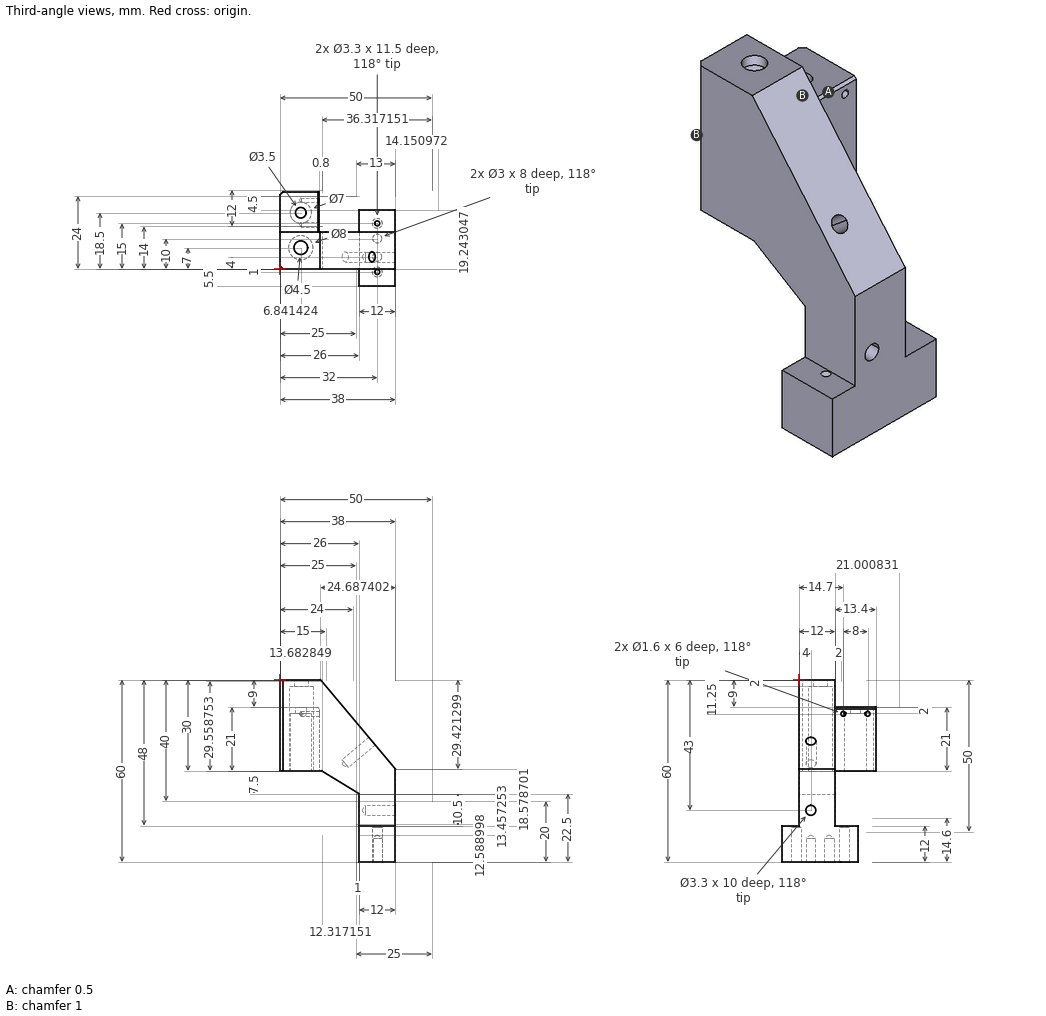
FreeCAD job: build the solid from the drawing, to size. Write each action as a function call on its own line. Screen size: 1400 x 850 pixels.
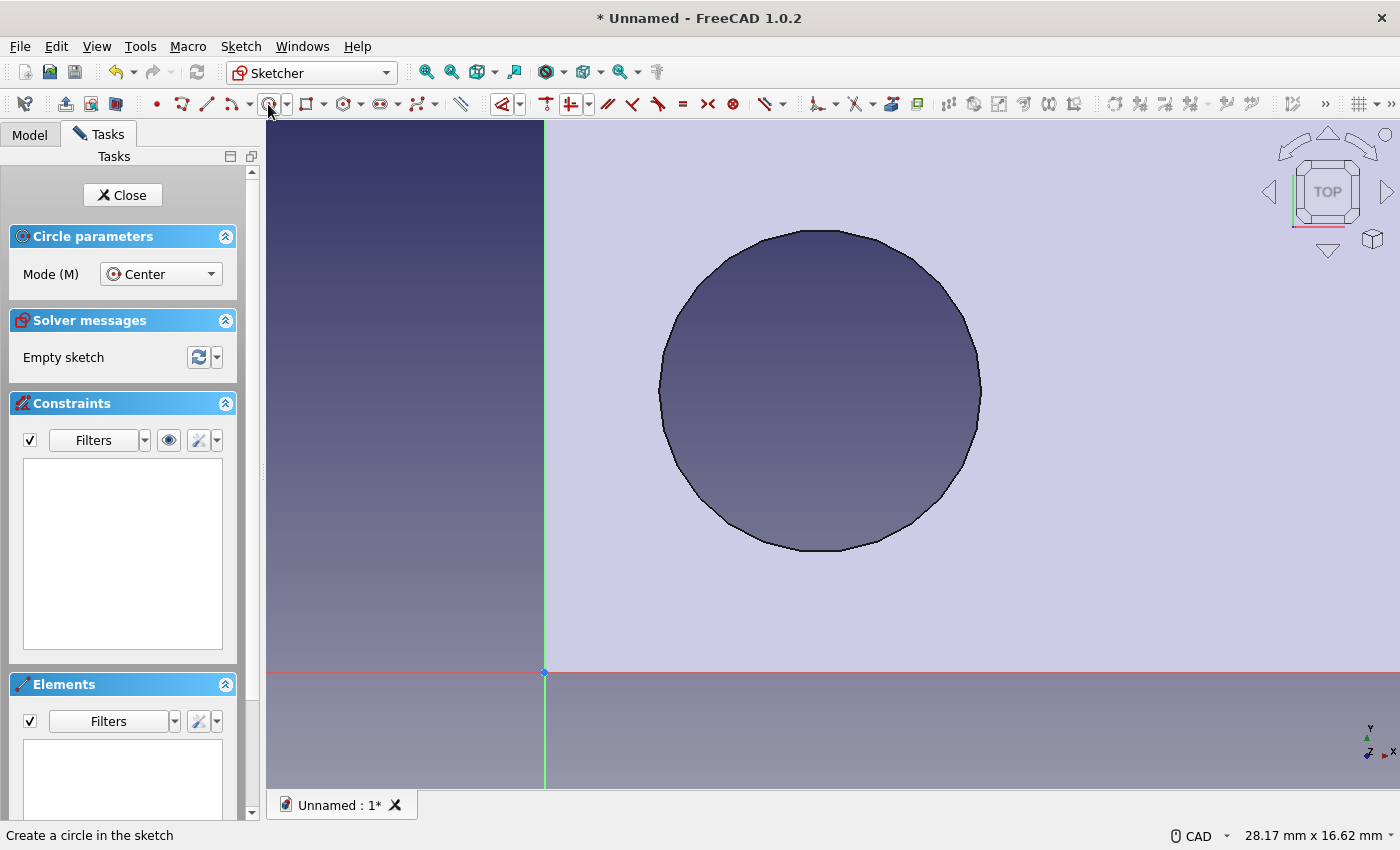
click(820, 391)
click(934, 277)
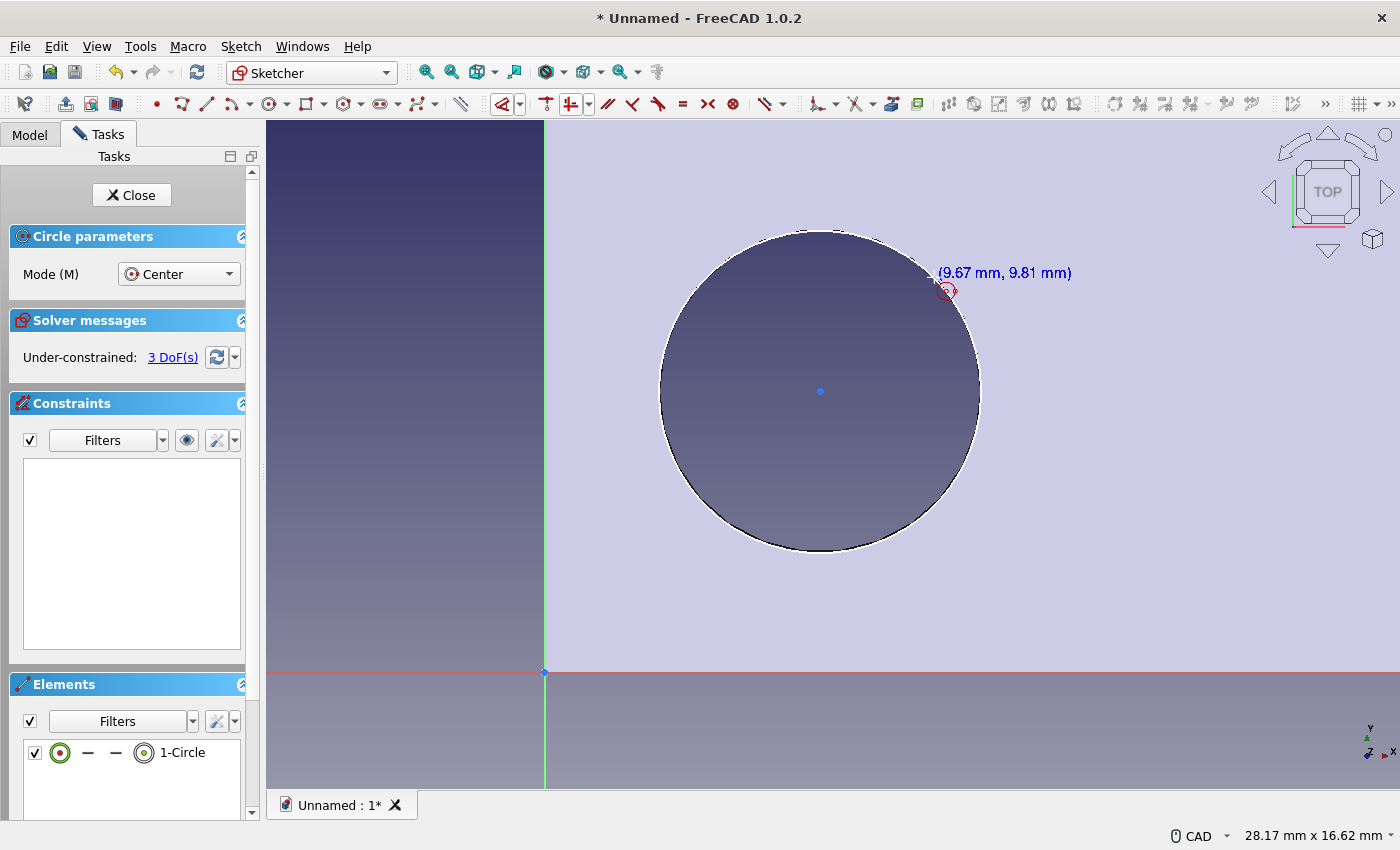
click(820, 392)
click(884, 327)
key(Escape)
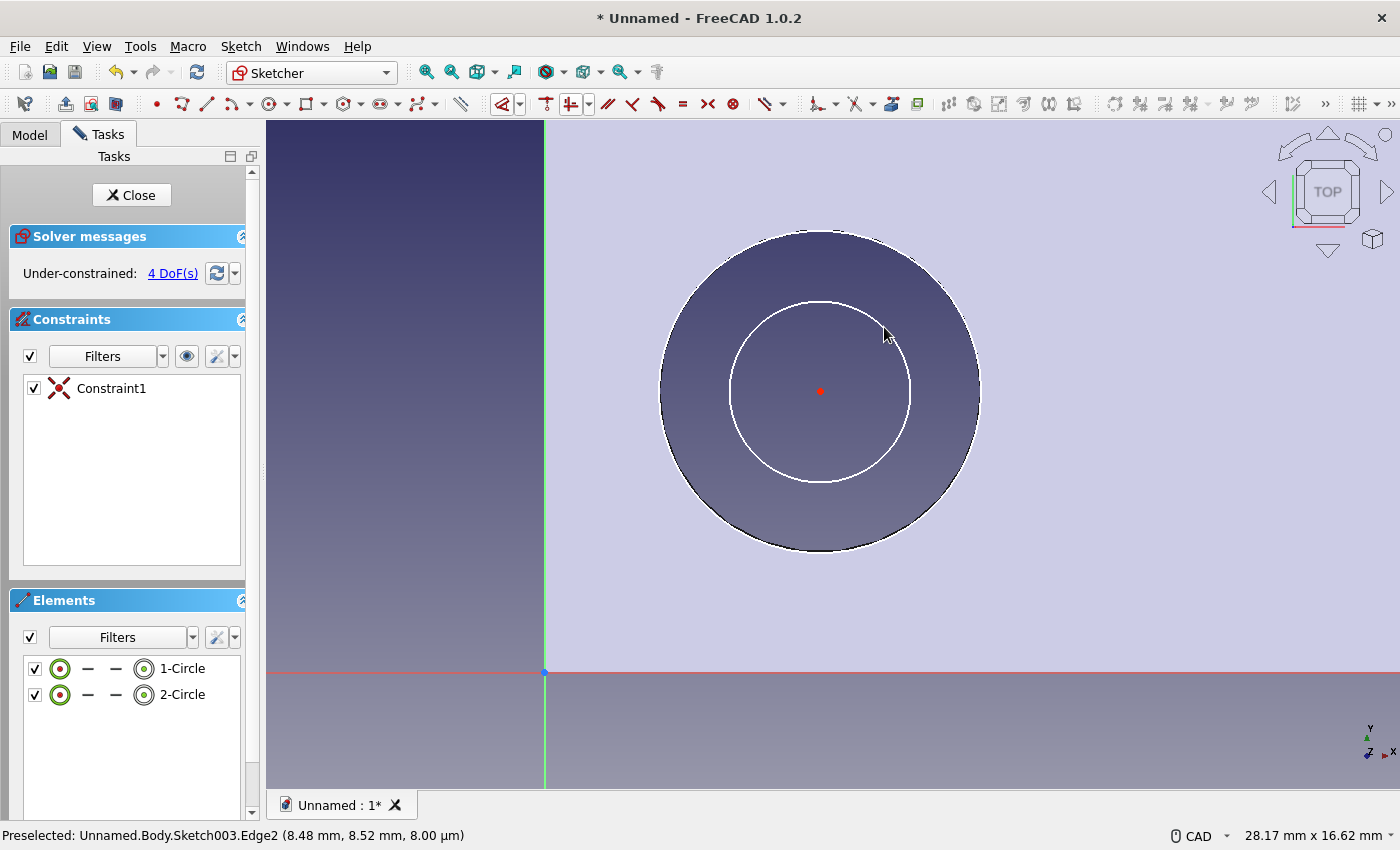
click(934, 278)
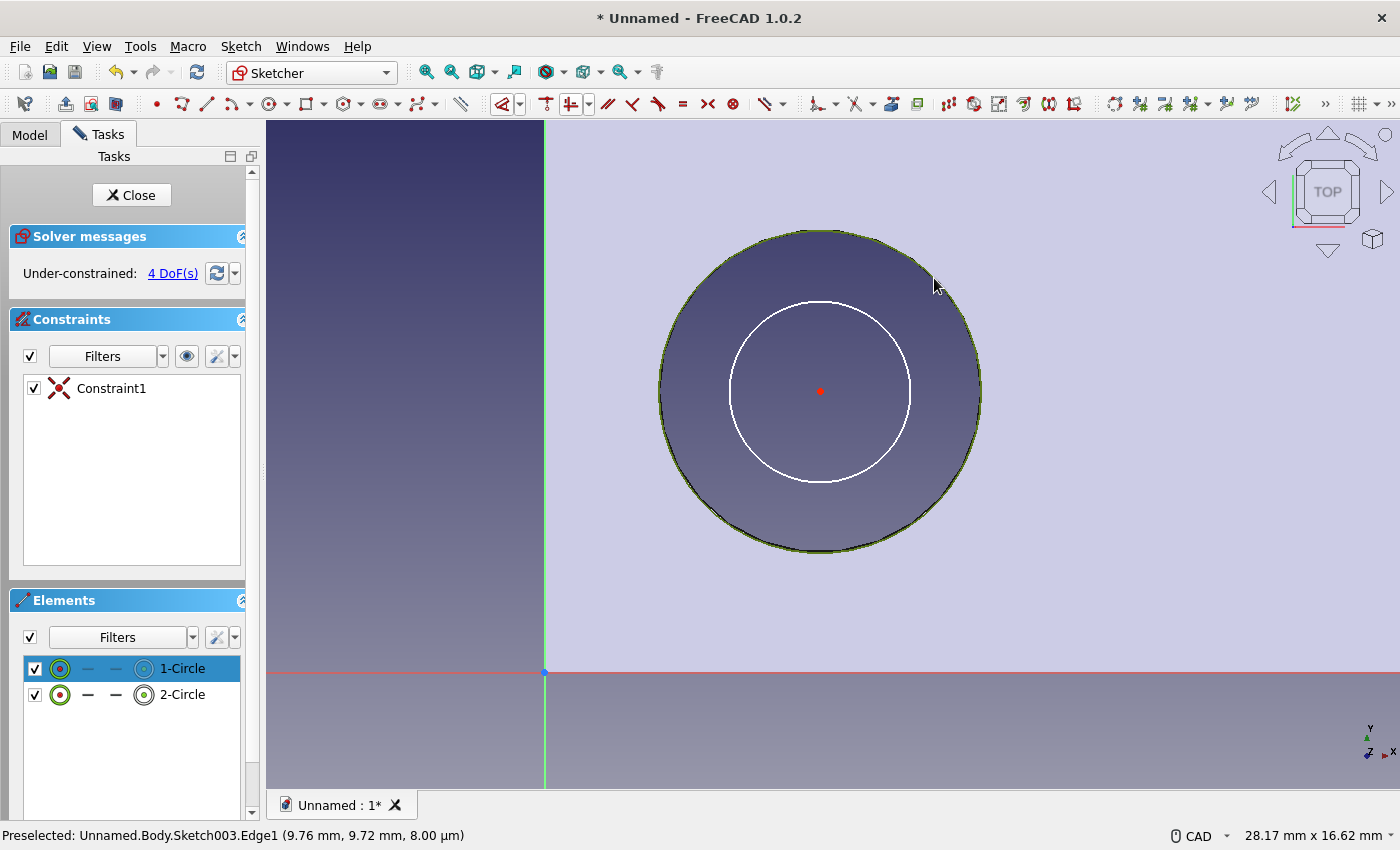
click(520, 104)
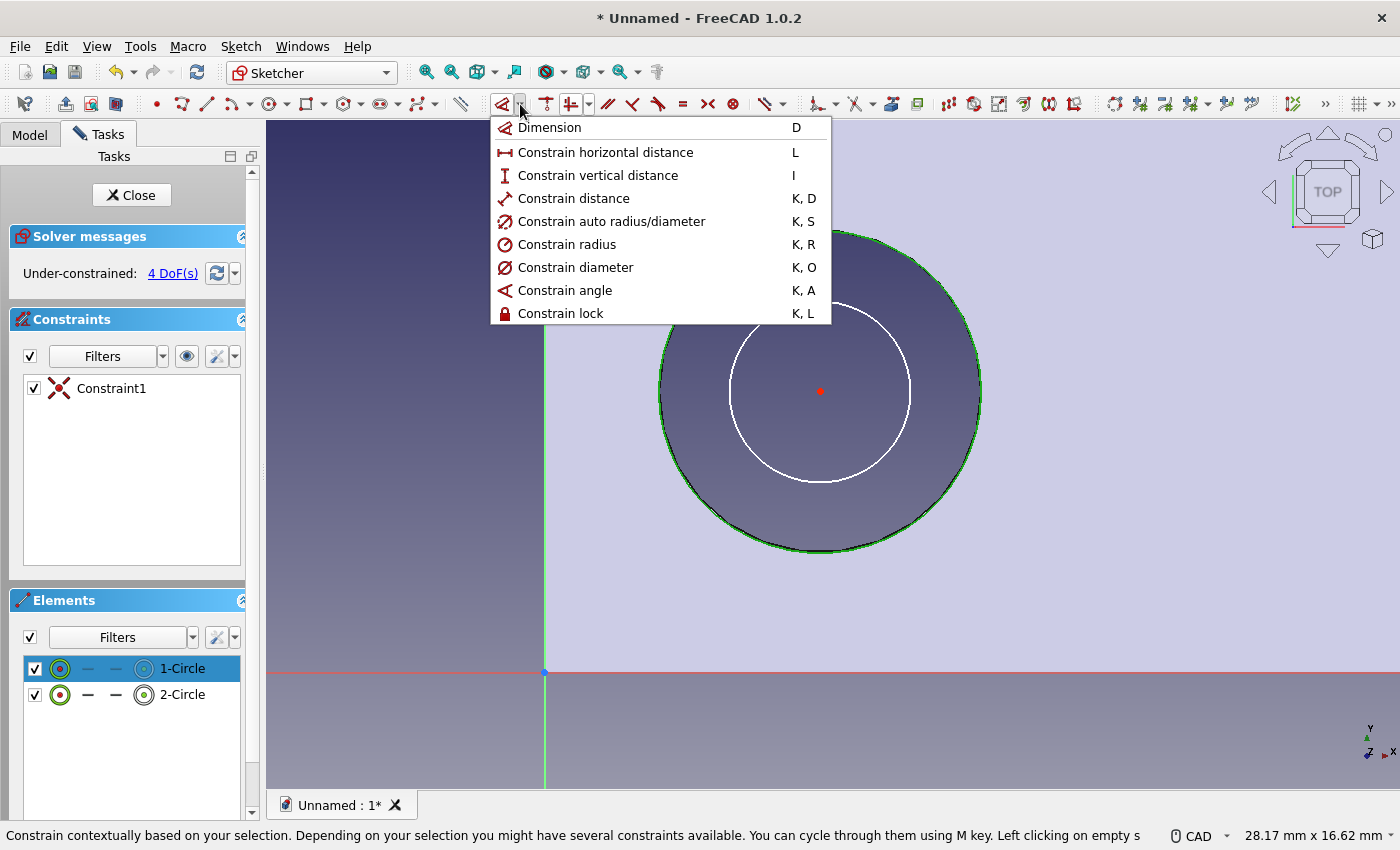
click(661, 268)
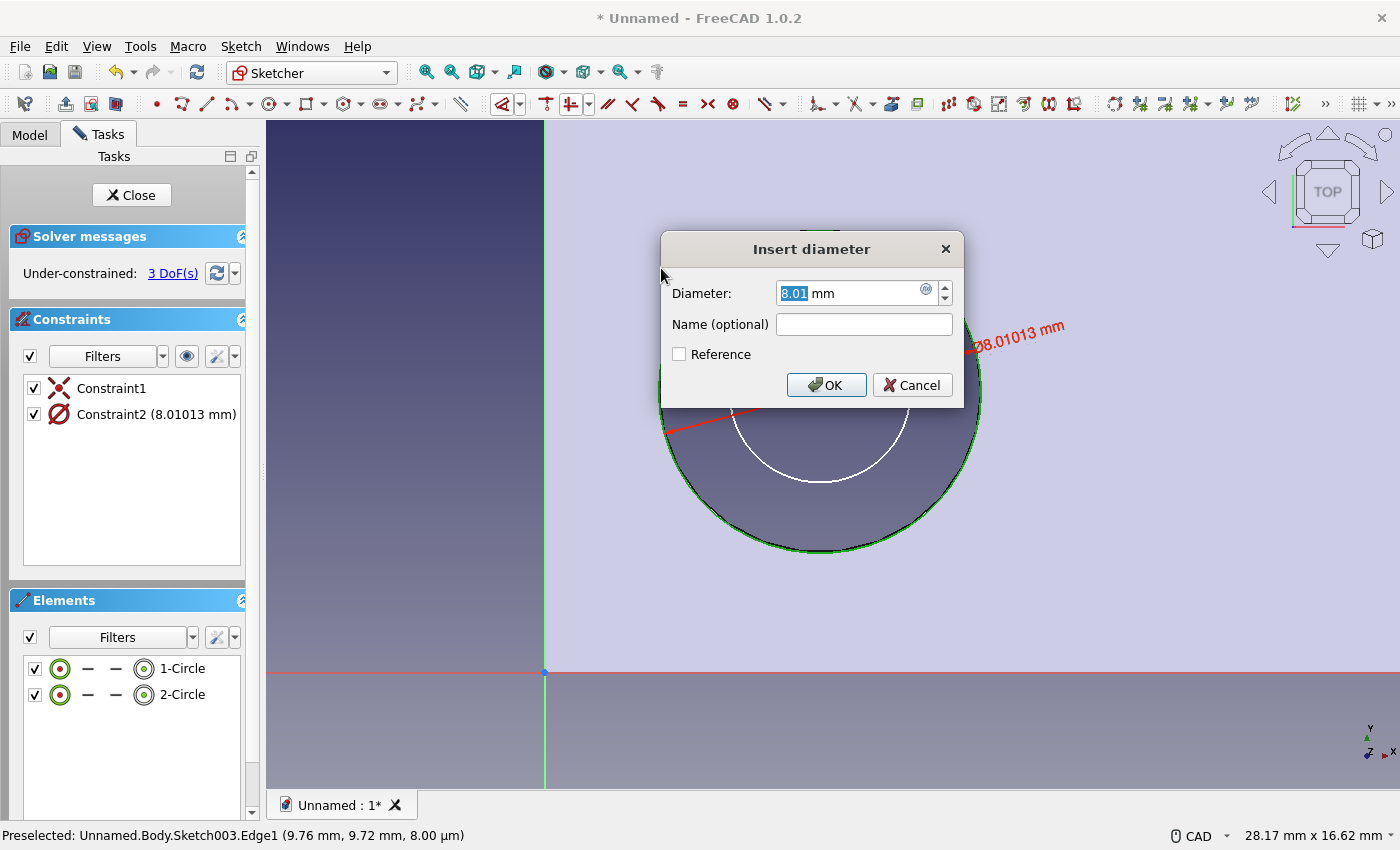
text(8)
key(Return)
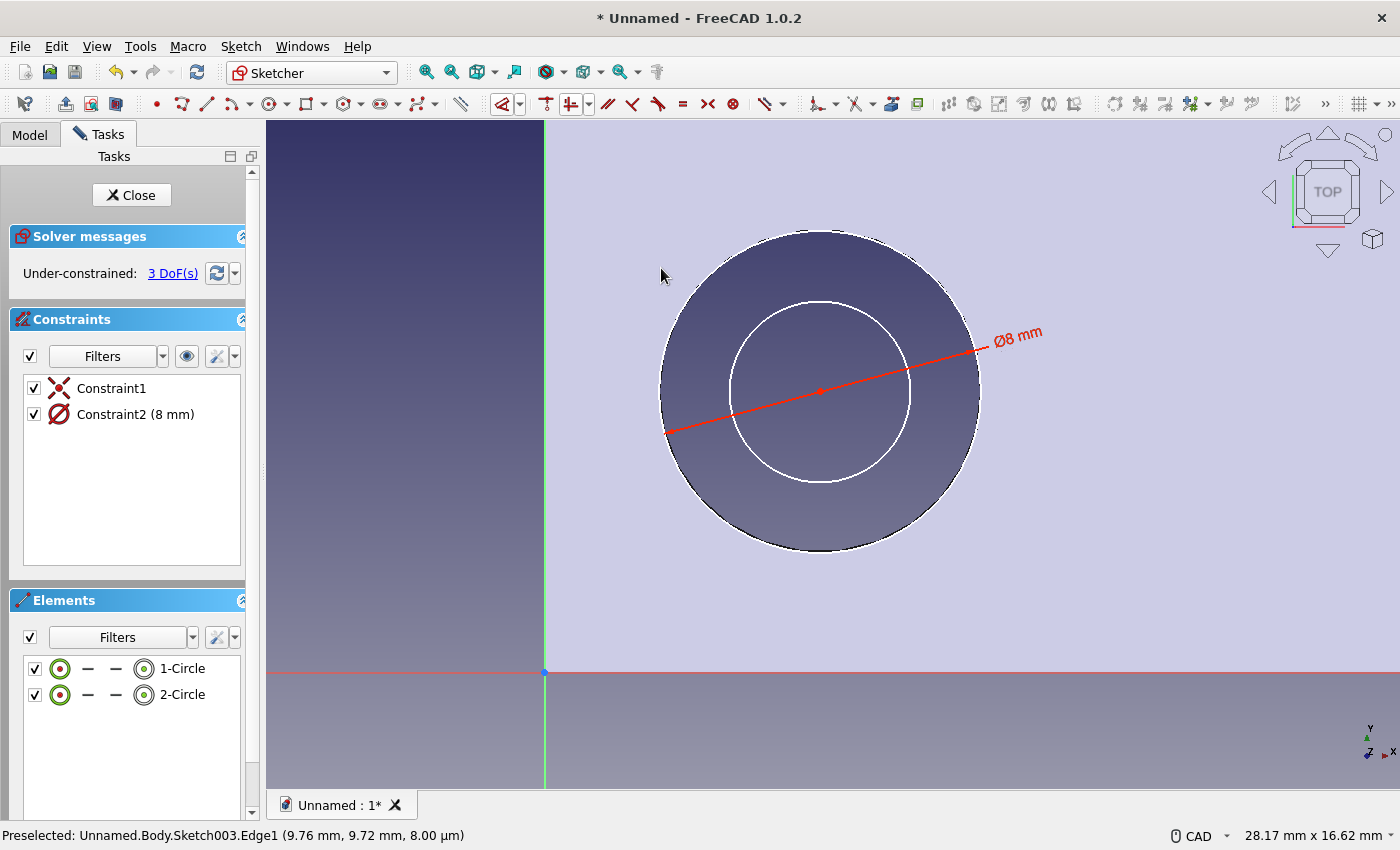
click(884, 328)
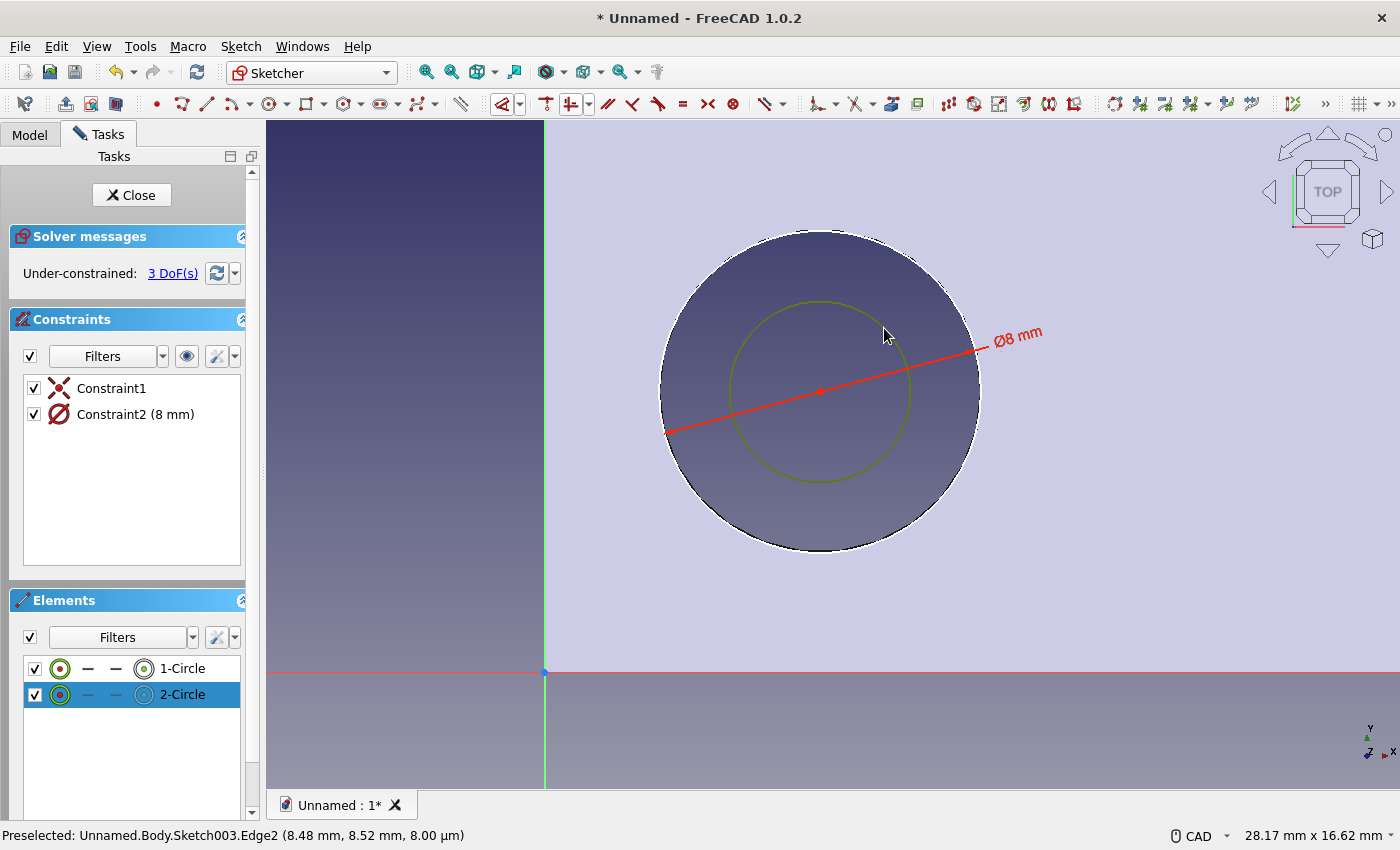
click(520, 104)